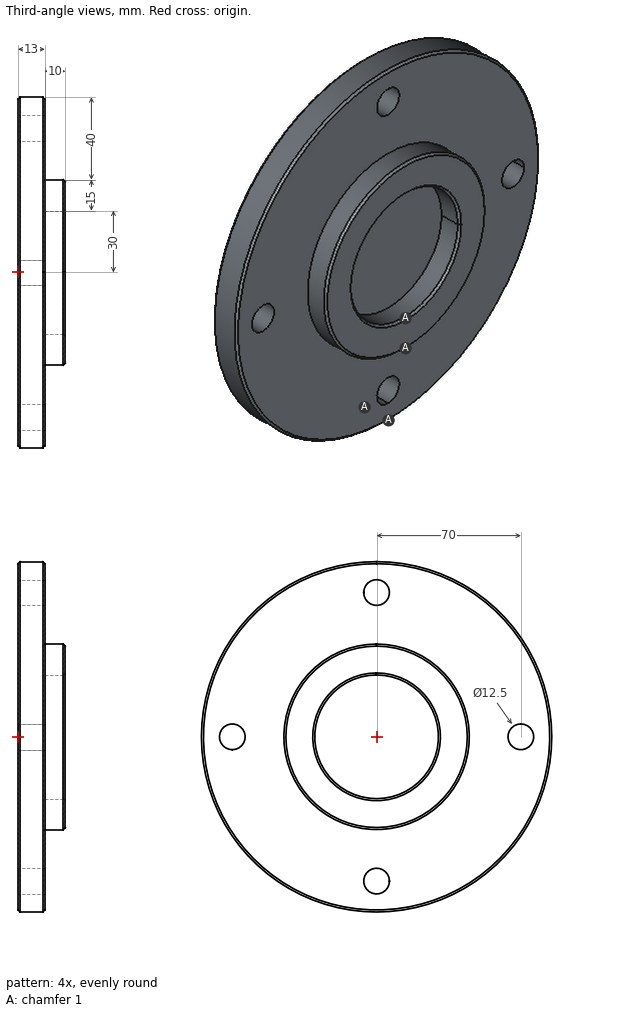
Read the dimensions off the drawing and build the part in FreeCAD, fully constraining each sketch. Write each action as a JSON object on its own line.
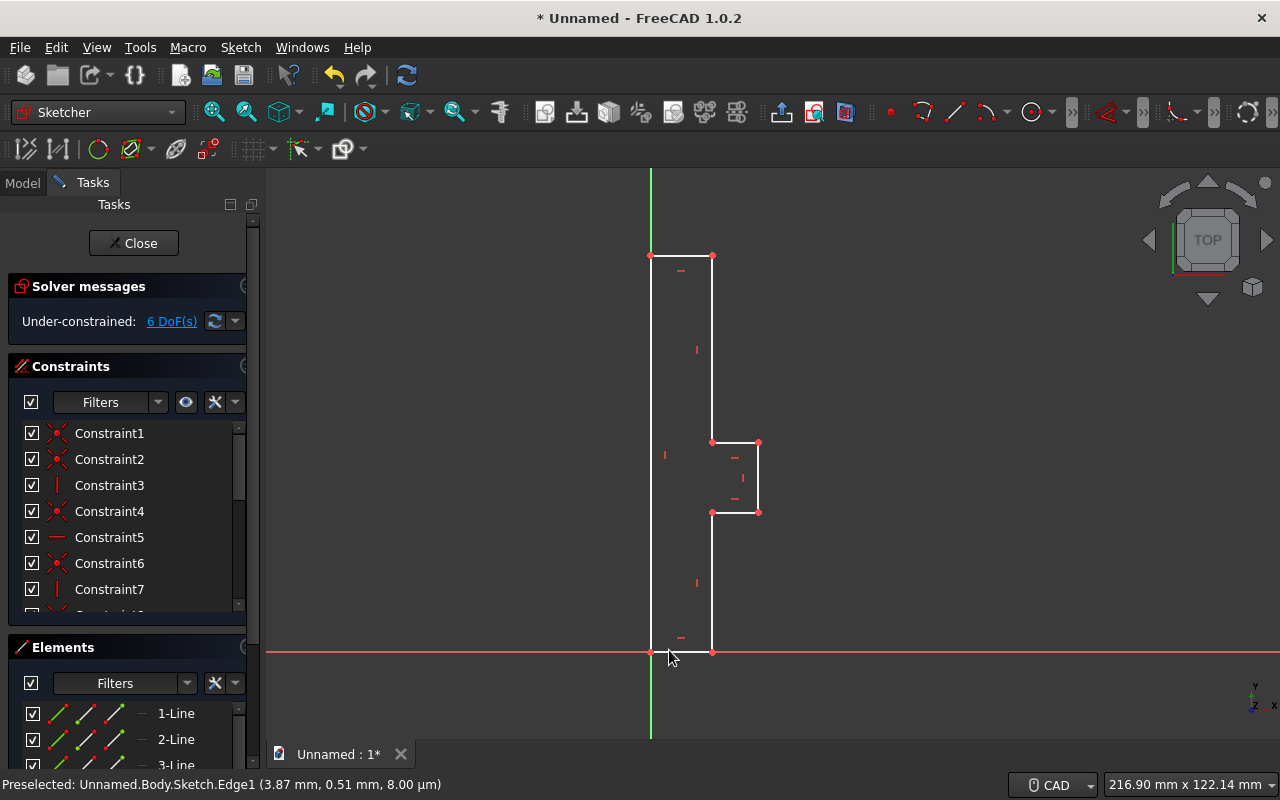
{"action": "key", "text": "d"}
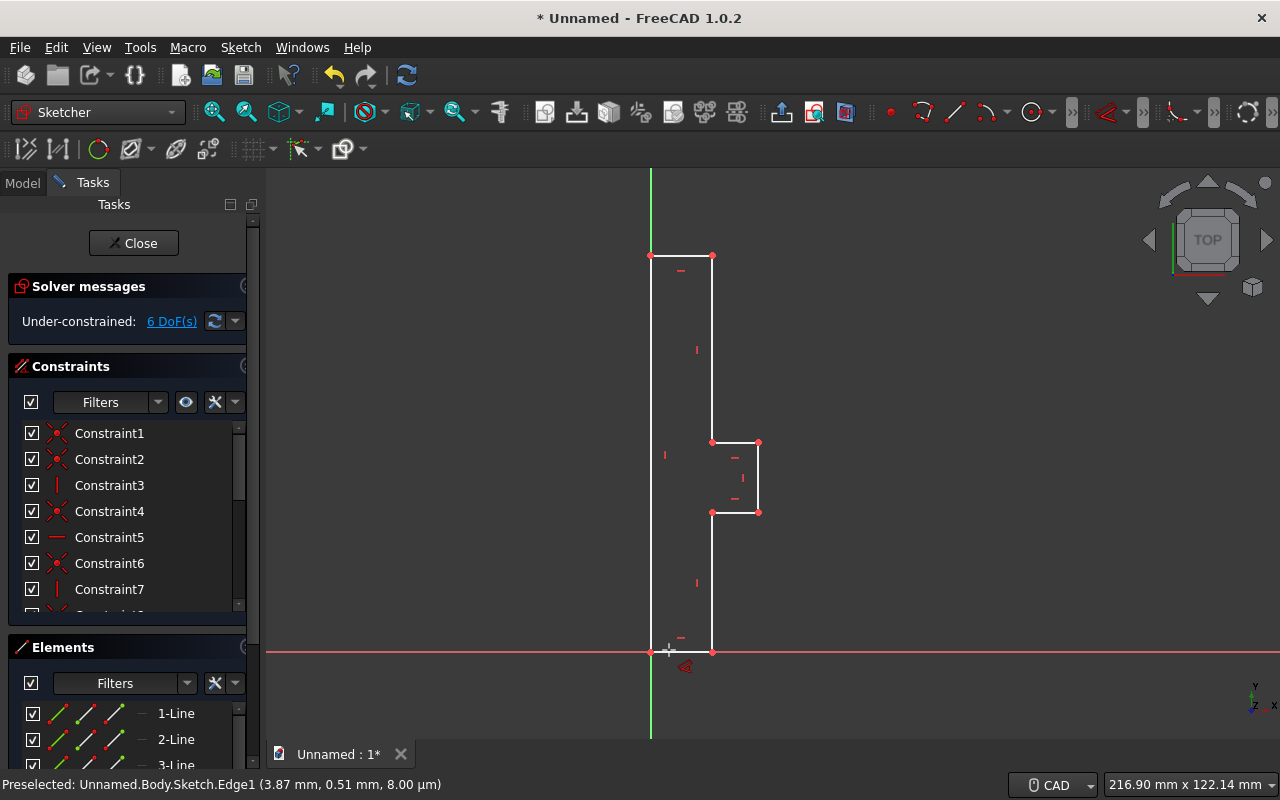
{"action": "left_click", "coordinate": [669, 652]}
{"action": "left_click", "coordinate": [681, 686]}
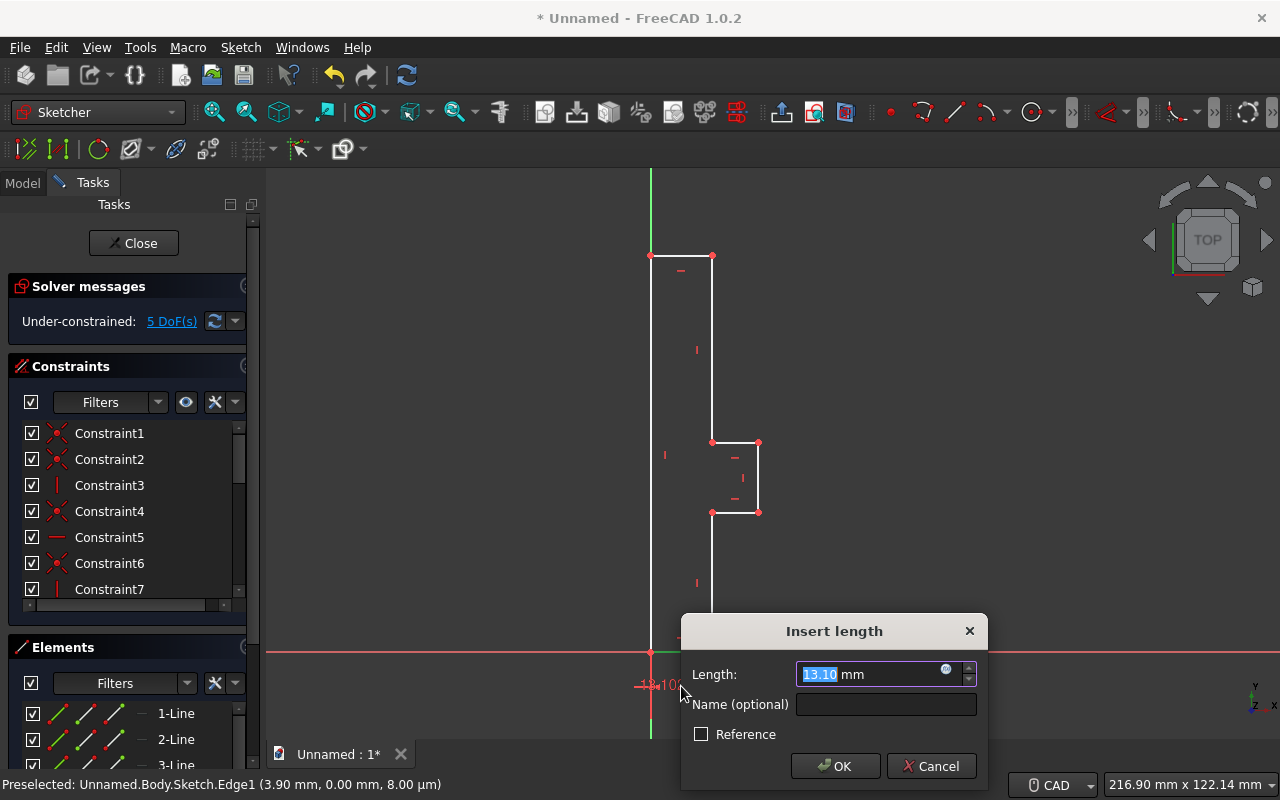
{"action": "type", "text": "13"}
{"action": "key", "text": "Return"}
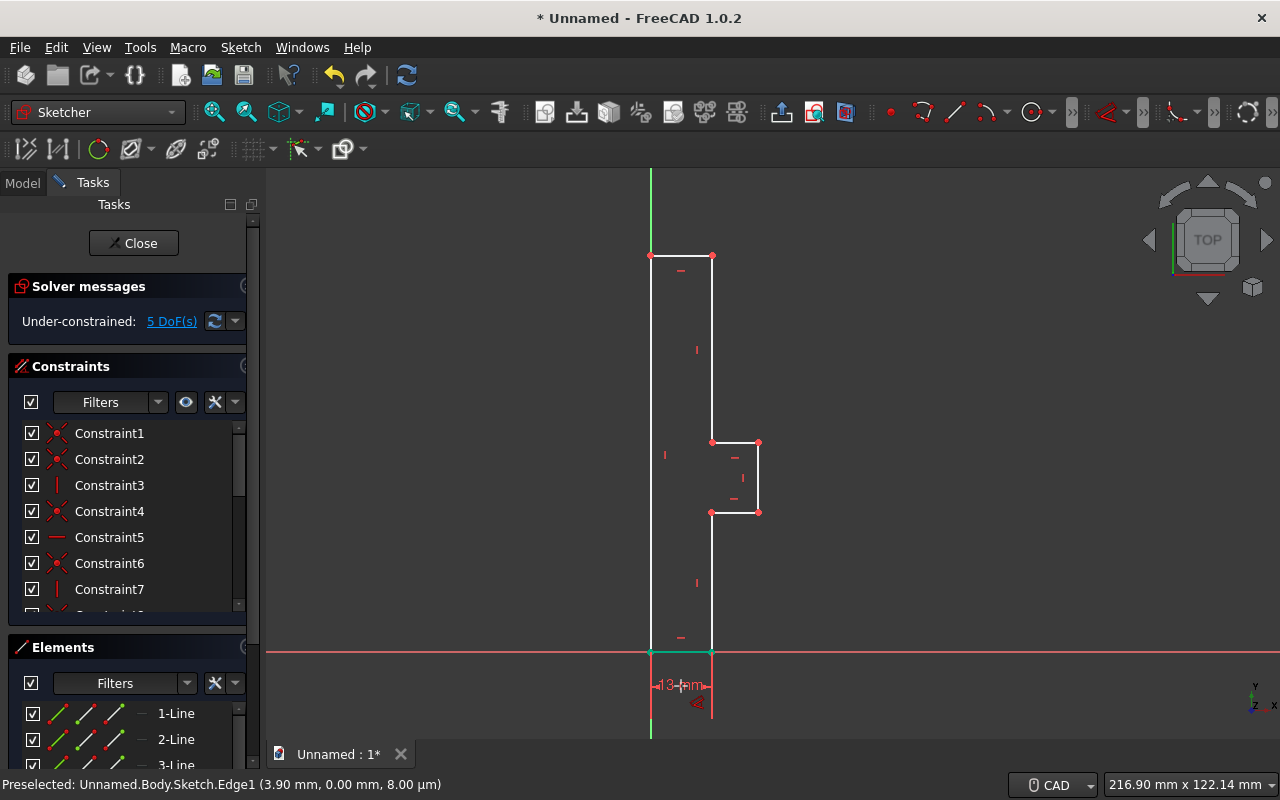
{"action": "left_click", "coordinate": [712, 610]}
{"action": "left_click", "coordinate": [746, 583]}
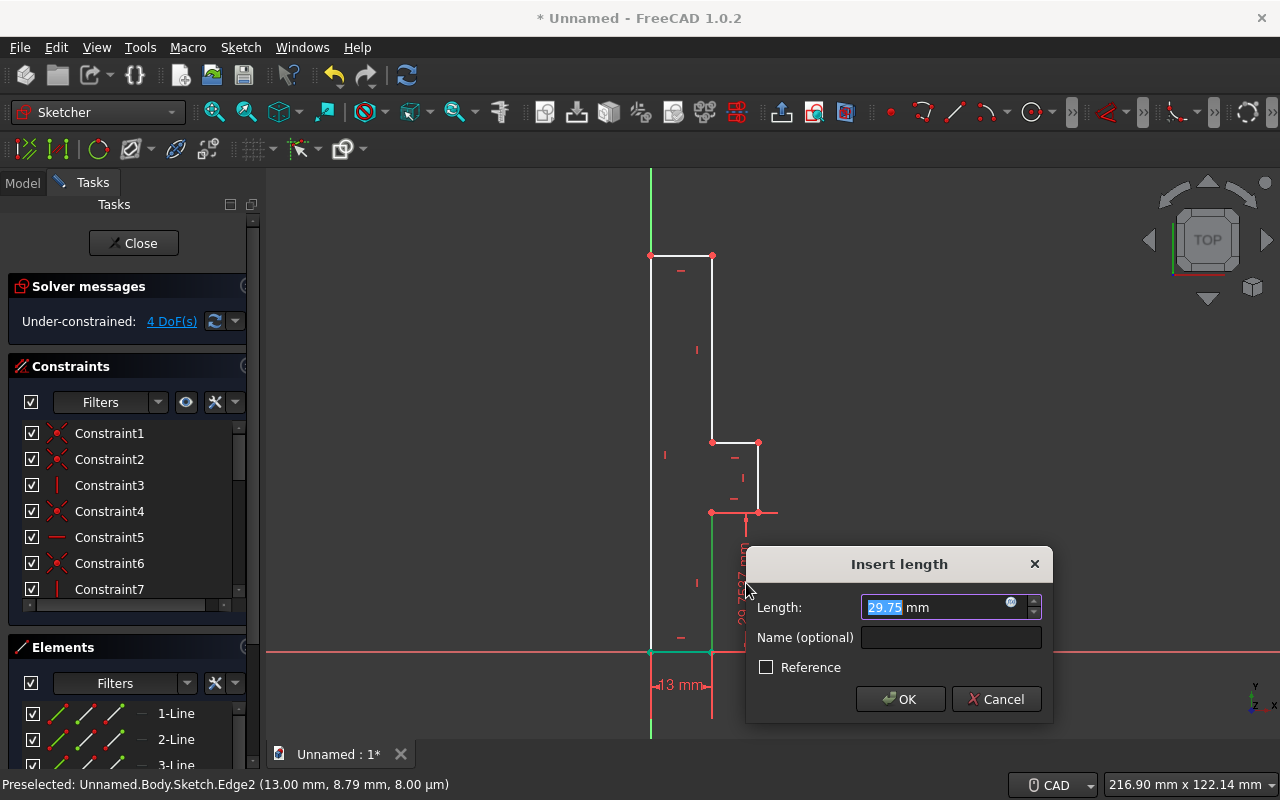
{"action": "type", "text": "30"}
{"action": "key", "text": "Return"}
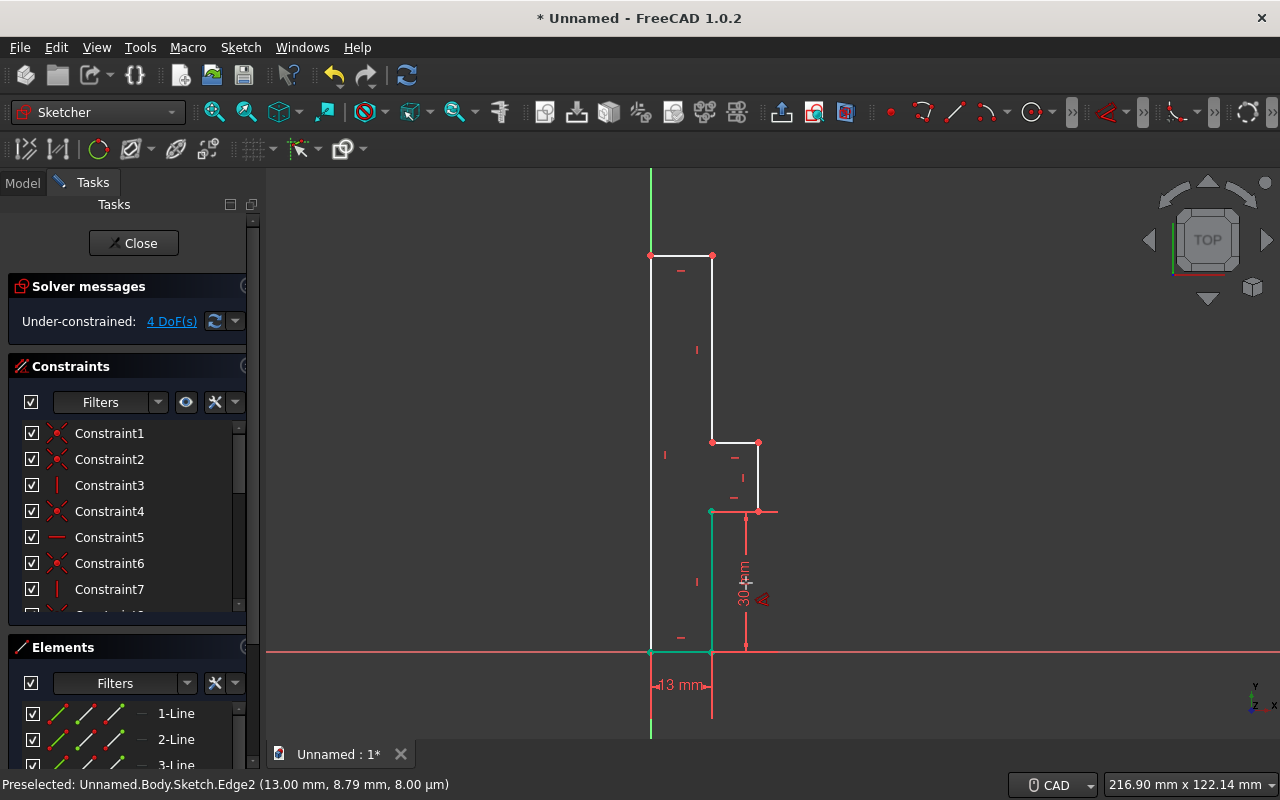
{"action": "left_click", "coordinate": [725, 512]}
{"action": "left_click", "coordinate": [735, 546]}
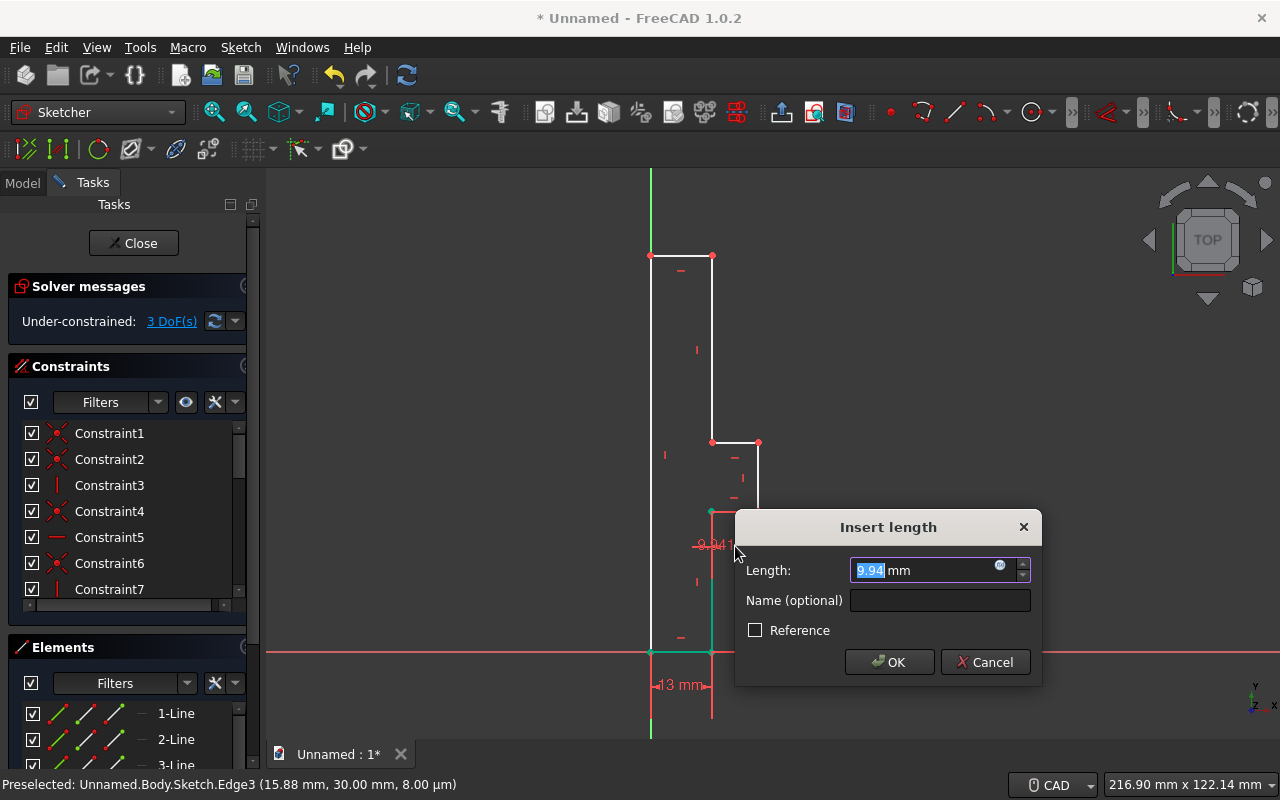
{"action": "type", "text": "10"}
{"action": "key", "text": "Return"}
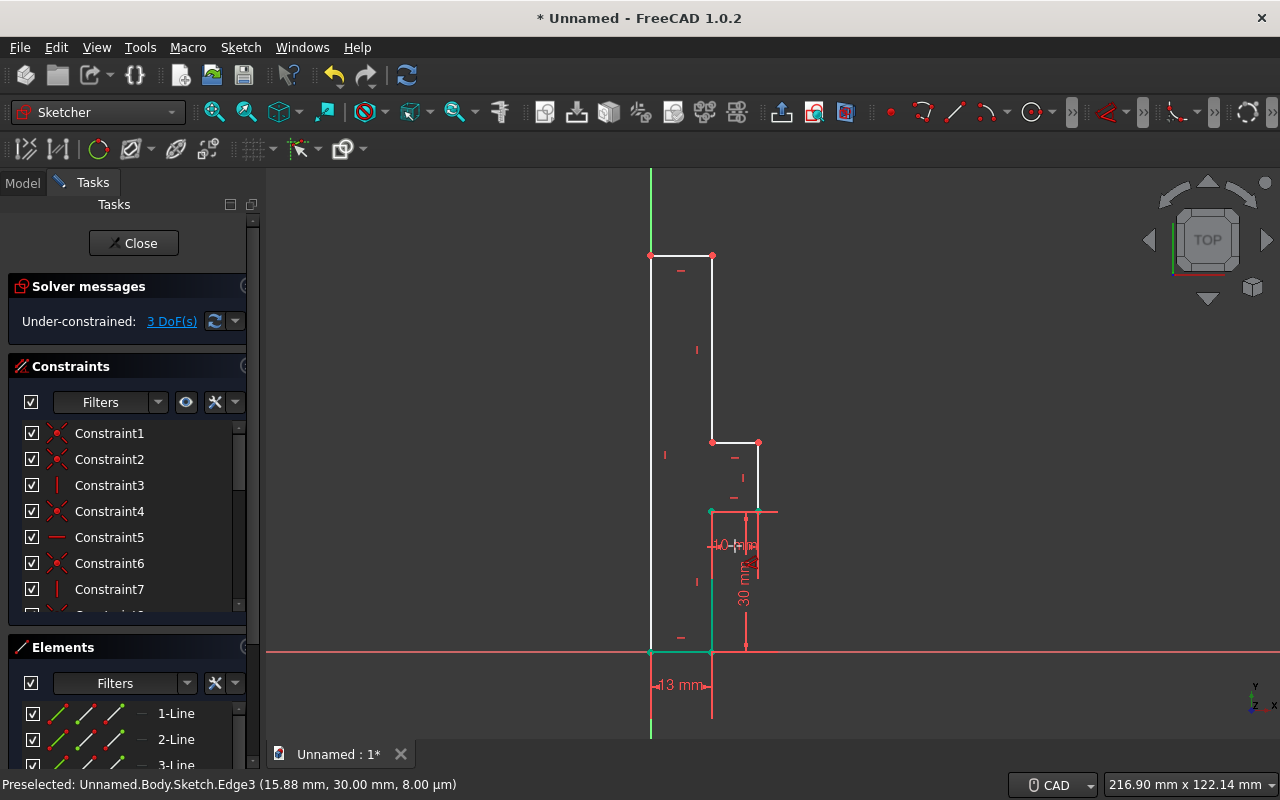
{"action": "left_click", "coordinate": [758, 491]}
{"action": "left_click", "coordinate": [792, 477]}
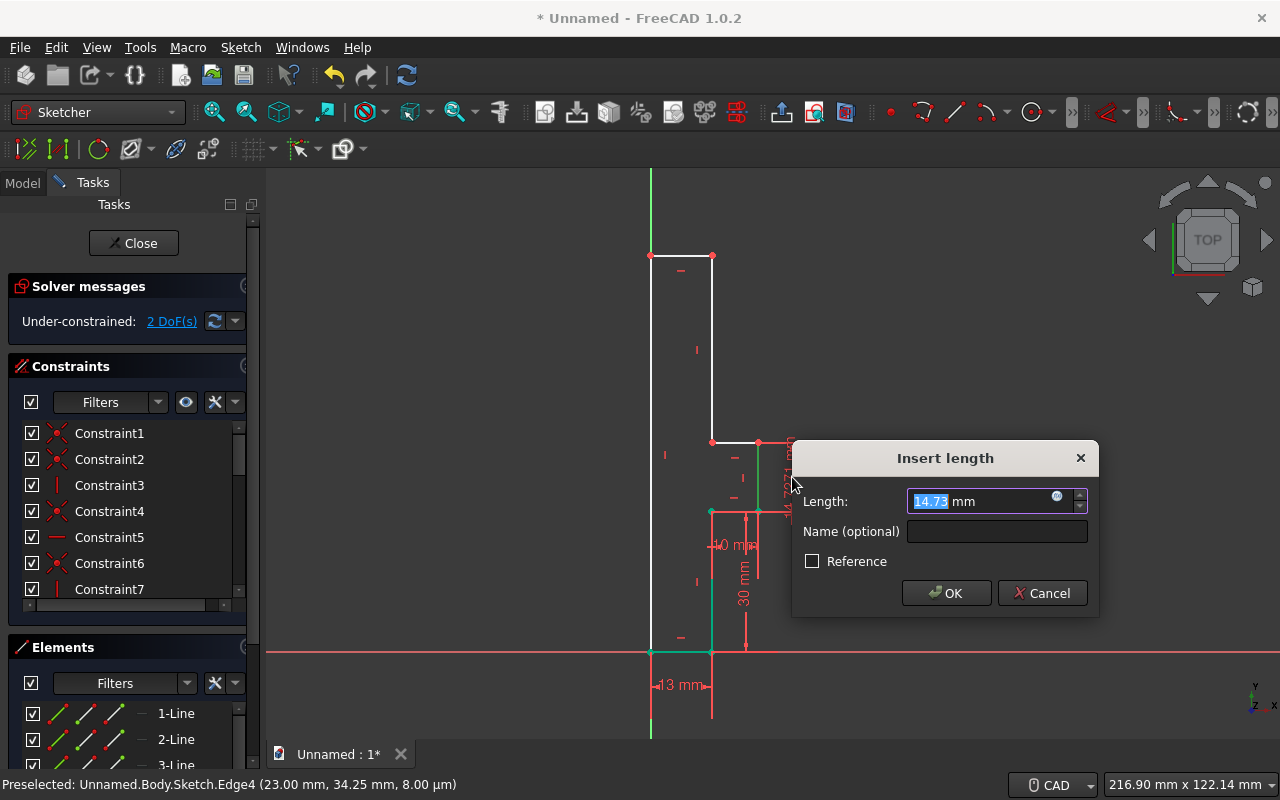
{"action": "type", "text": "15"}
{"action": "key", "text": "Return"}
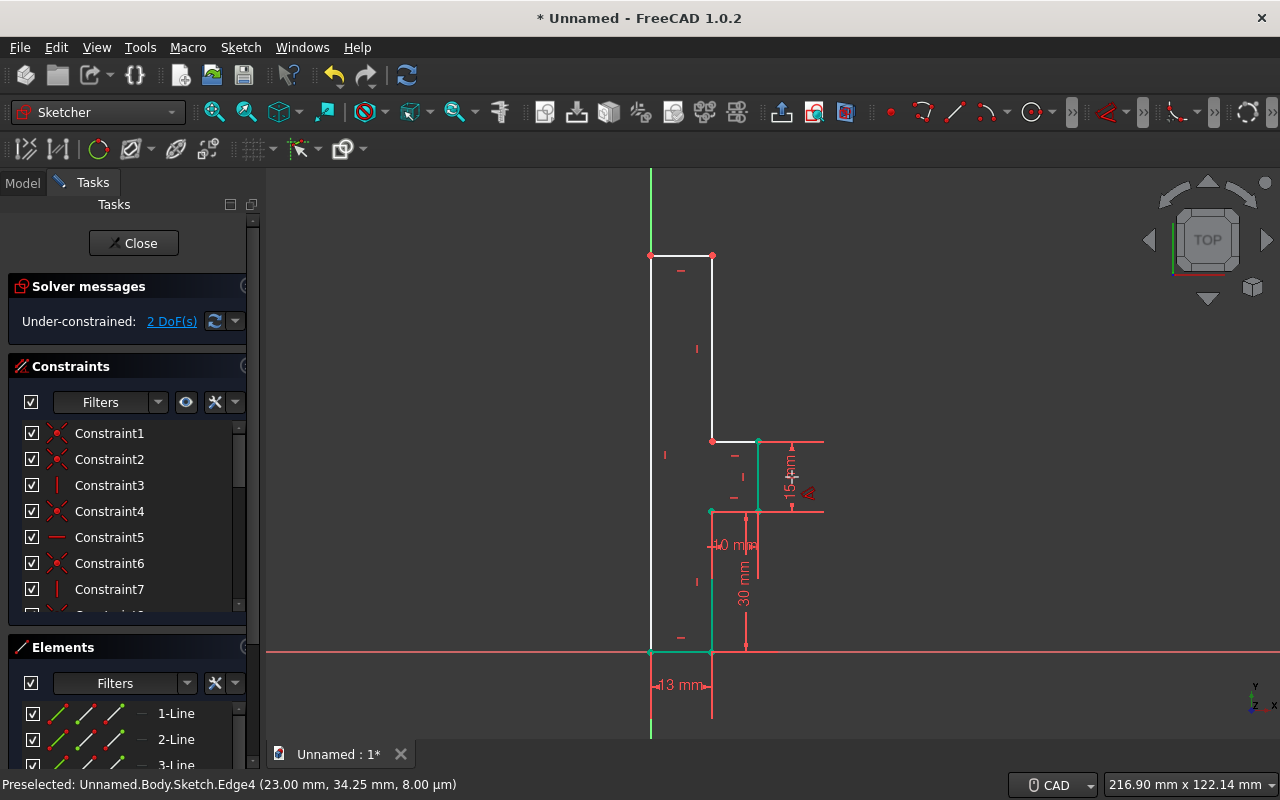
{"action": "left_click", "coordinate": [744, 442]}
{"action": "left_click", "coordinate": [735, 408]}